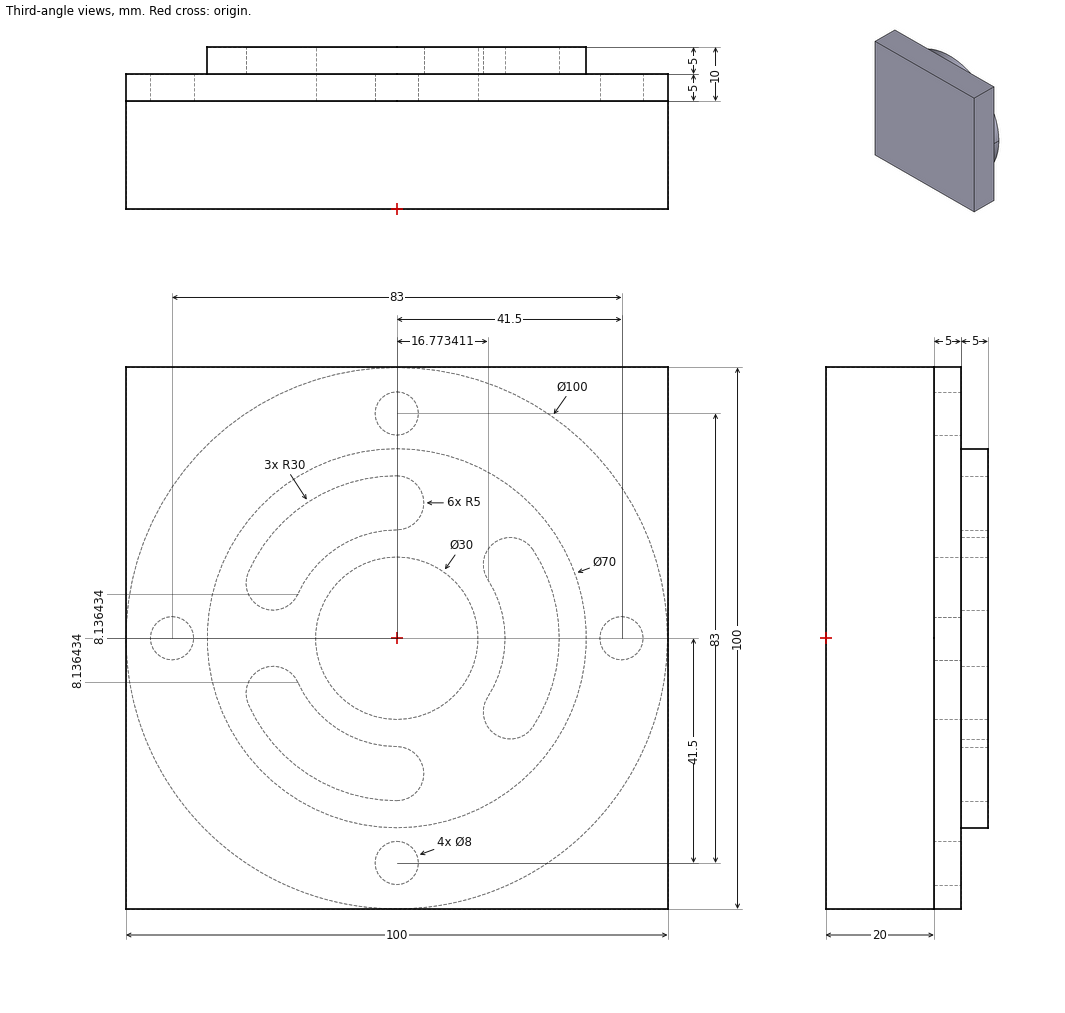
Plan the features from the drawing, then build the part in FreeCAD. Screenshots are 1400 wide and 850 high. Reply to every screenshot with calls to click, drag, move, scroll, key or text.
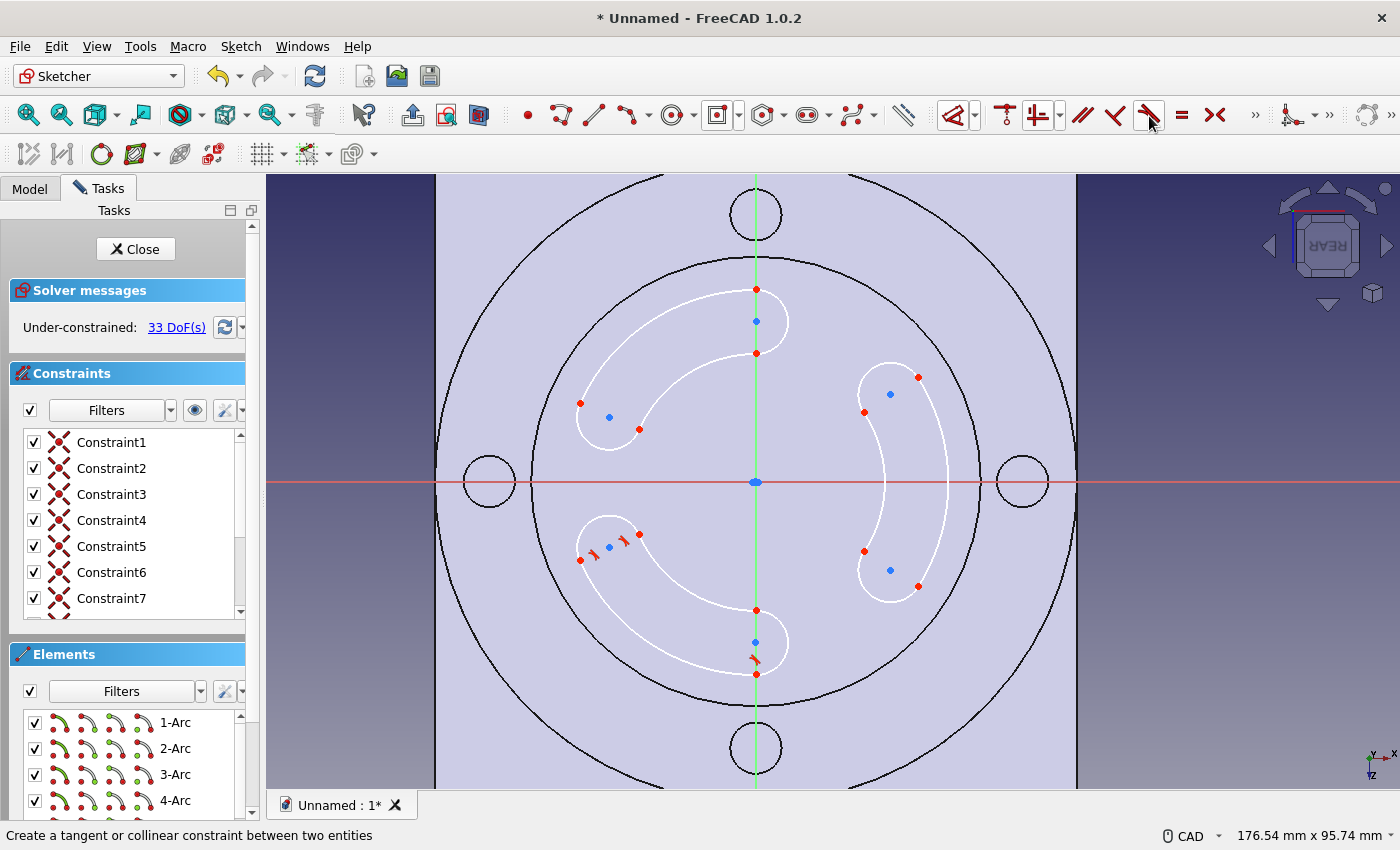
click(782, 662)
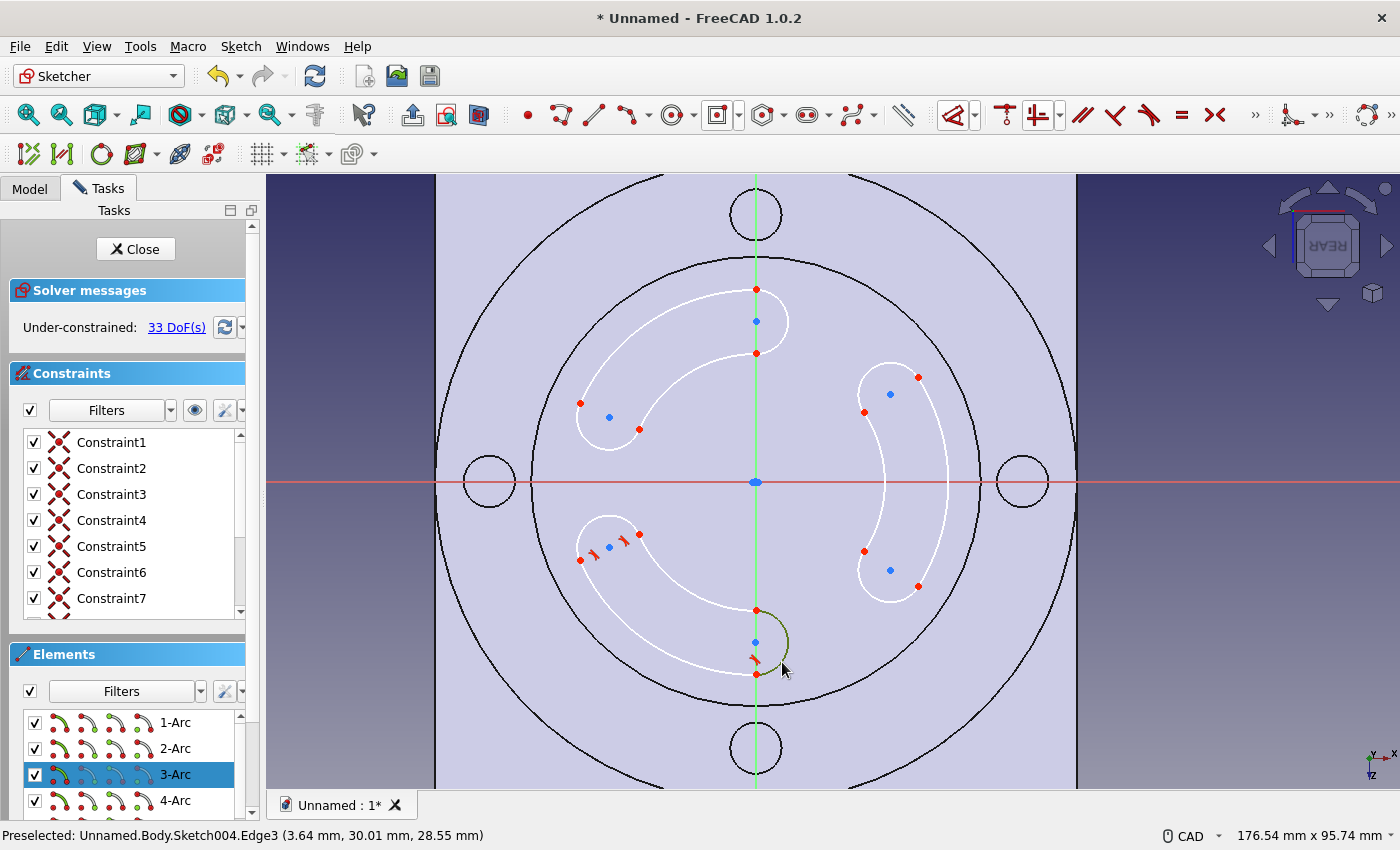
click(664, 571)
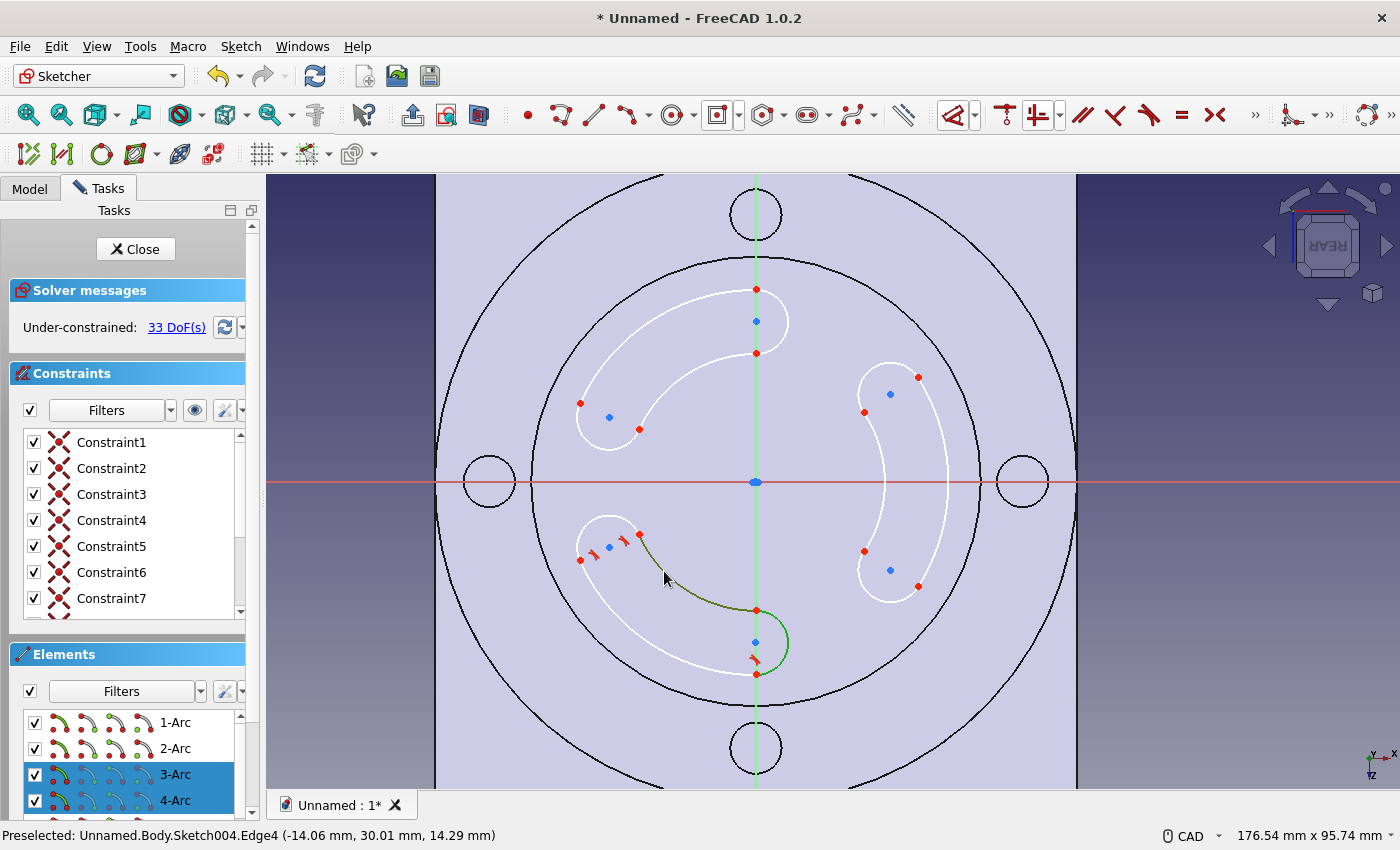
click(1149, 116)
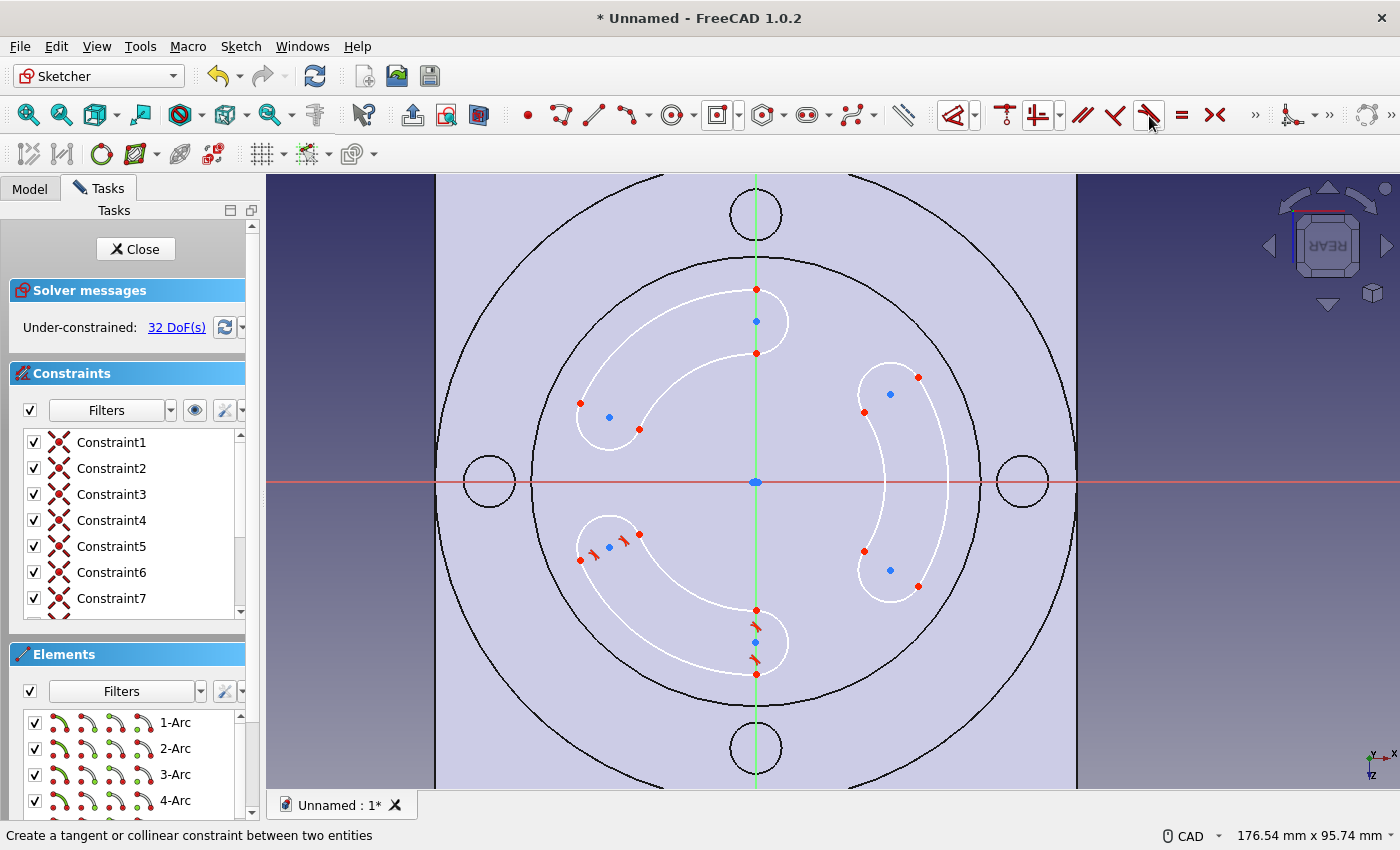
click(881, 512)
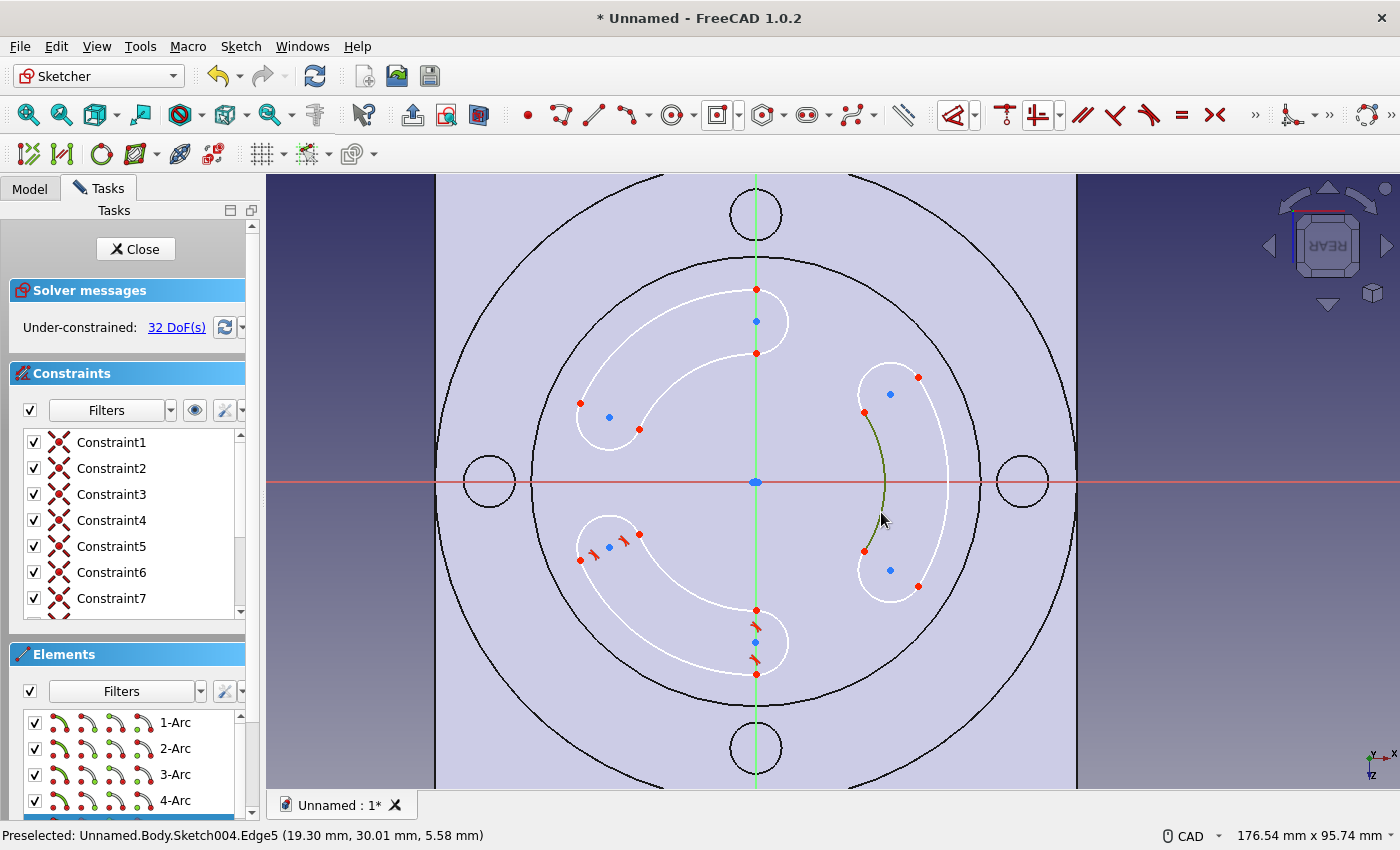
click(860, 581)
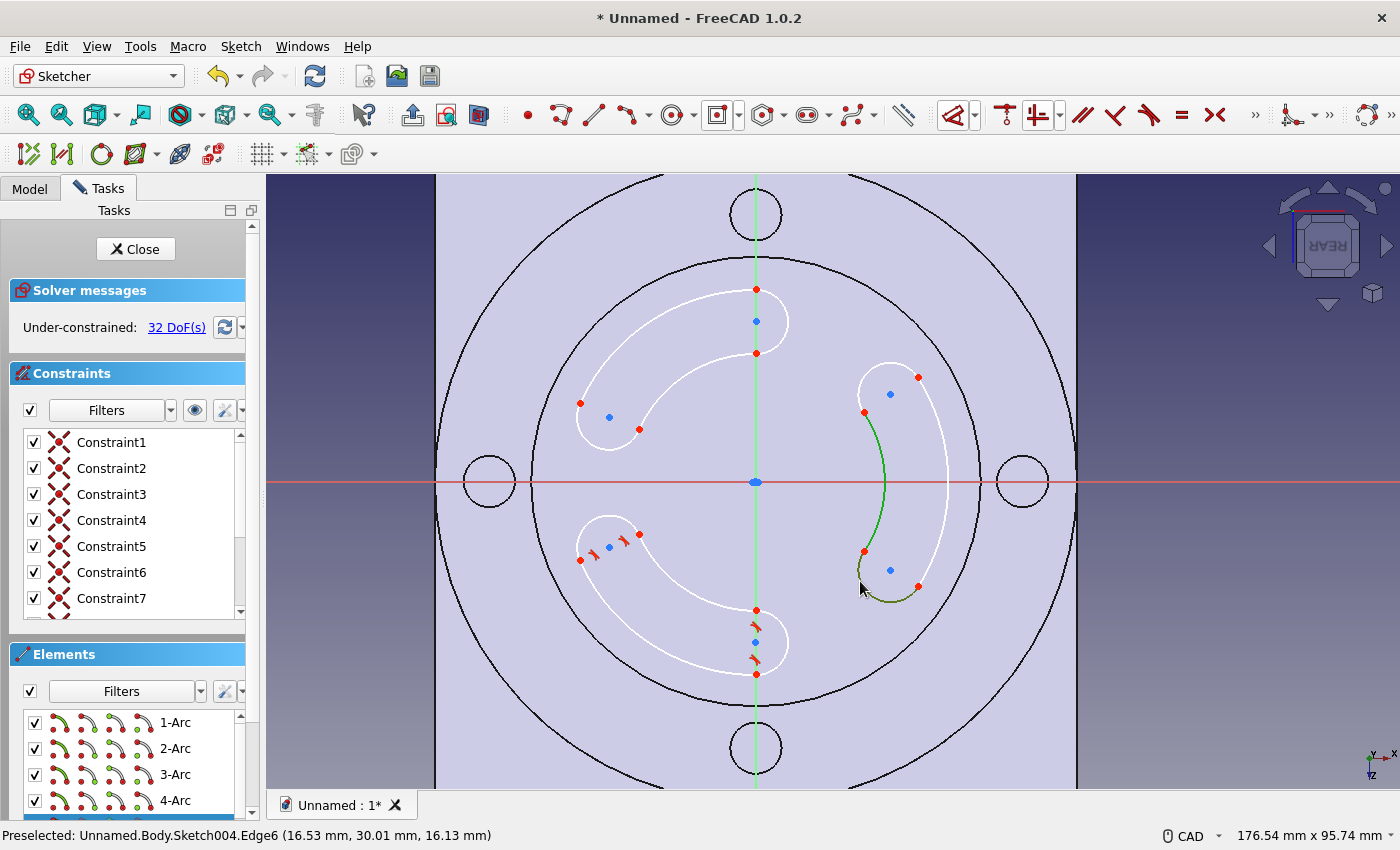
click(1149, 116)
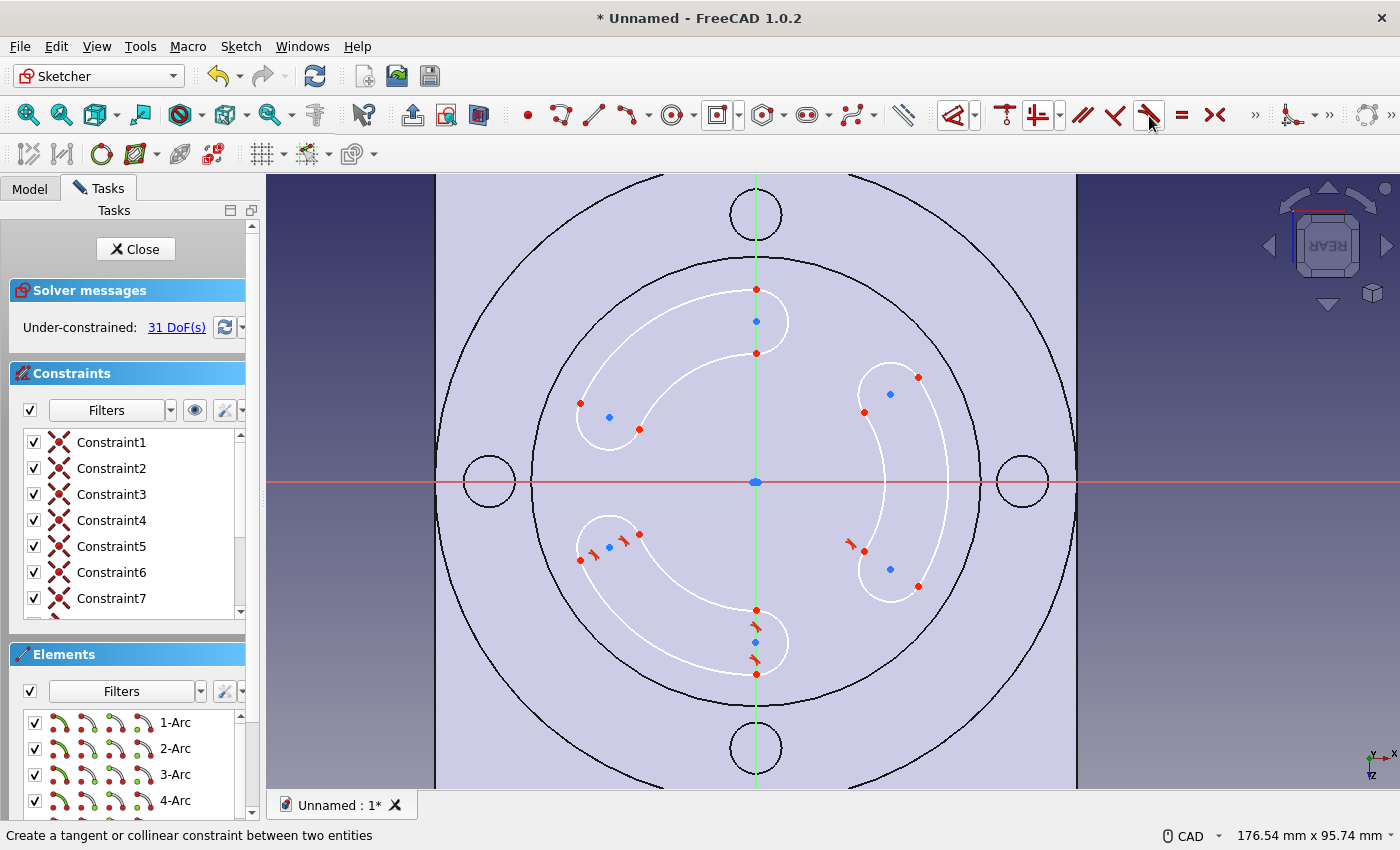
click(881, 512)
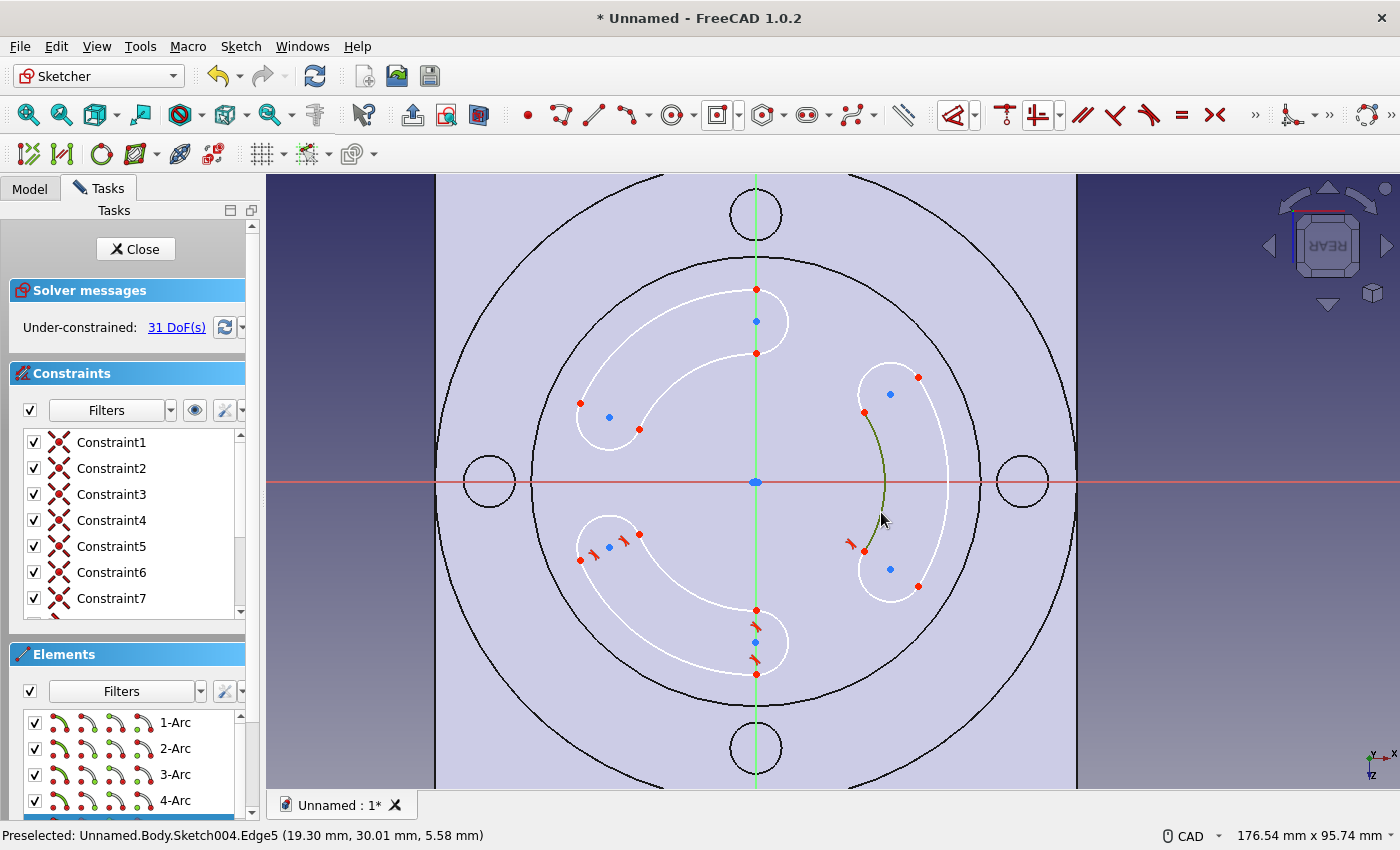
click(893, 363)